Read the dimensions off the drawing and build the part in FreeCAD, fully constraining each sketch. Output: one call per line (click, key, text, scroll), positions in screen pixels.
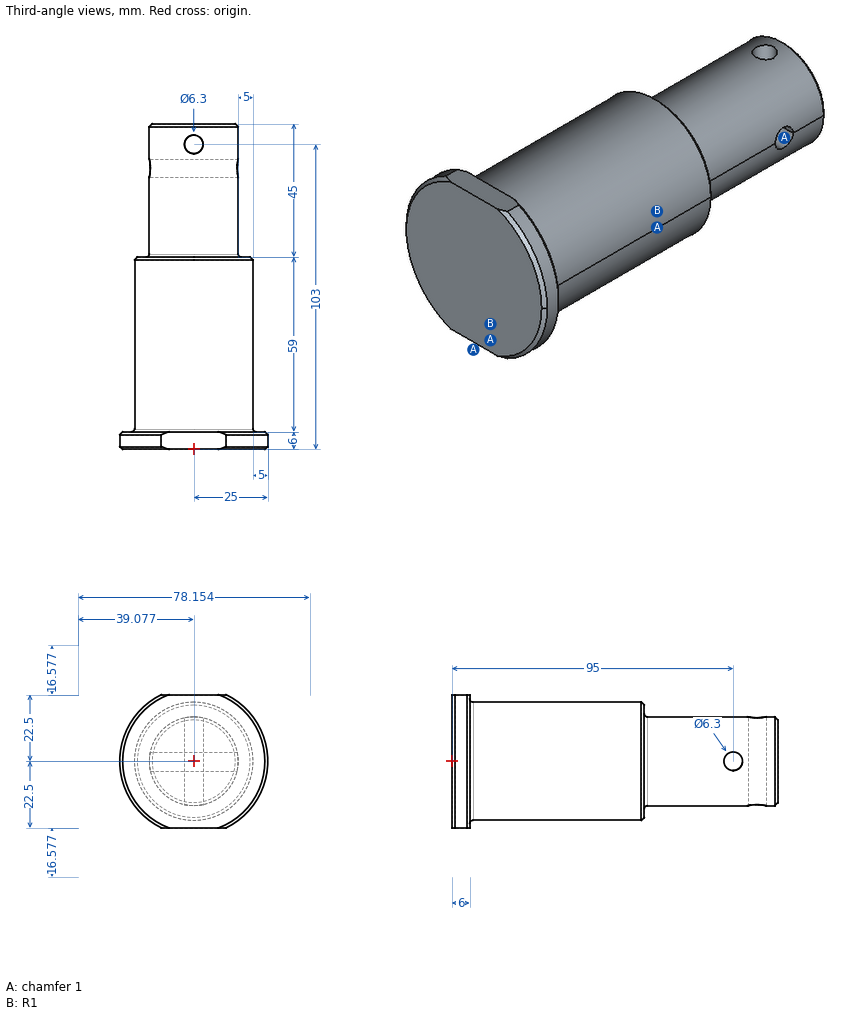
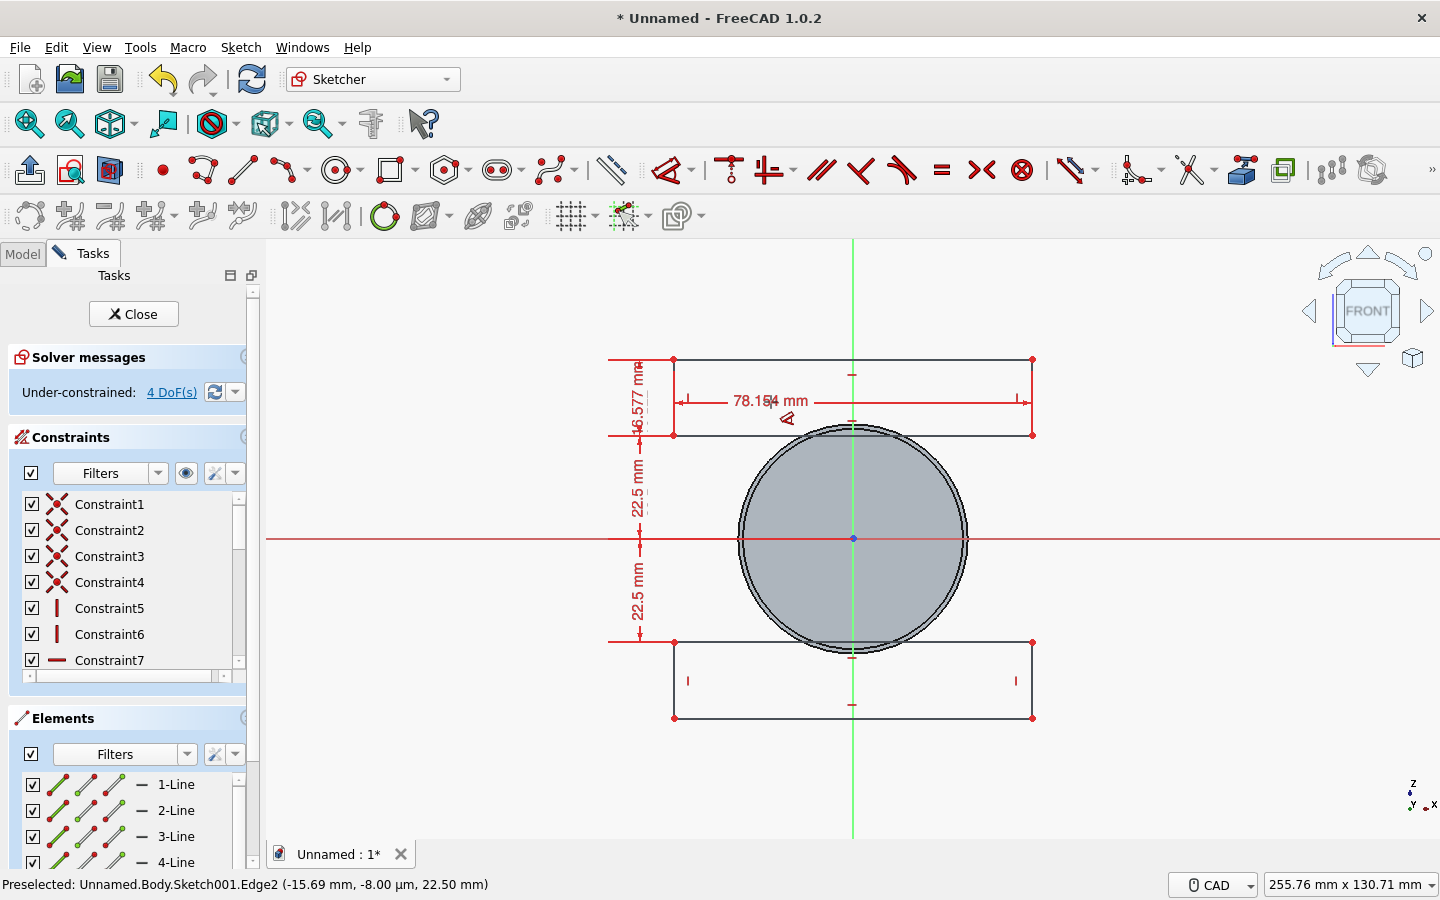
click(674, 665)
click(640, 681)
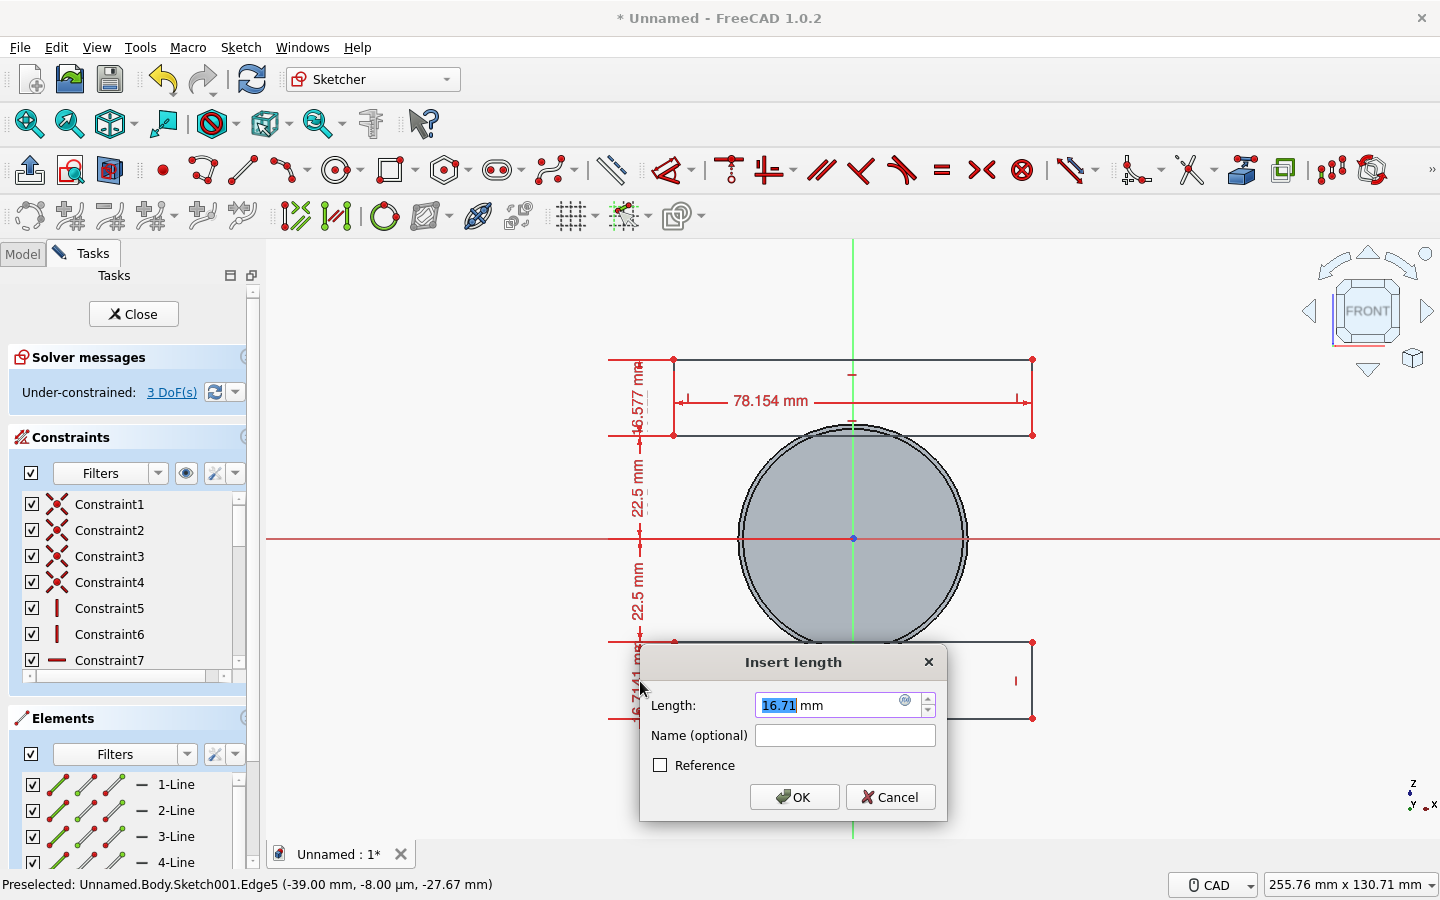
text(16.577)
key(Return)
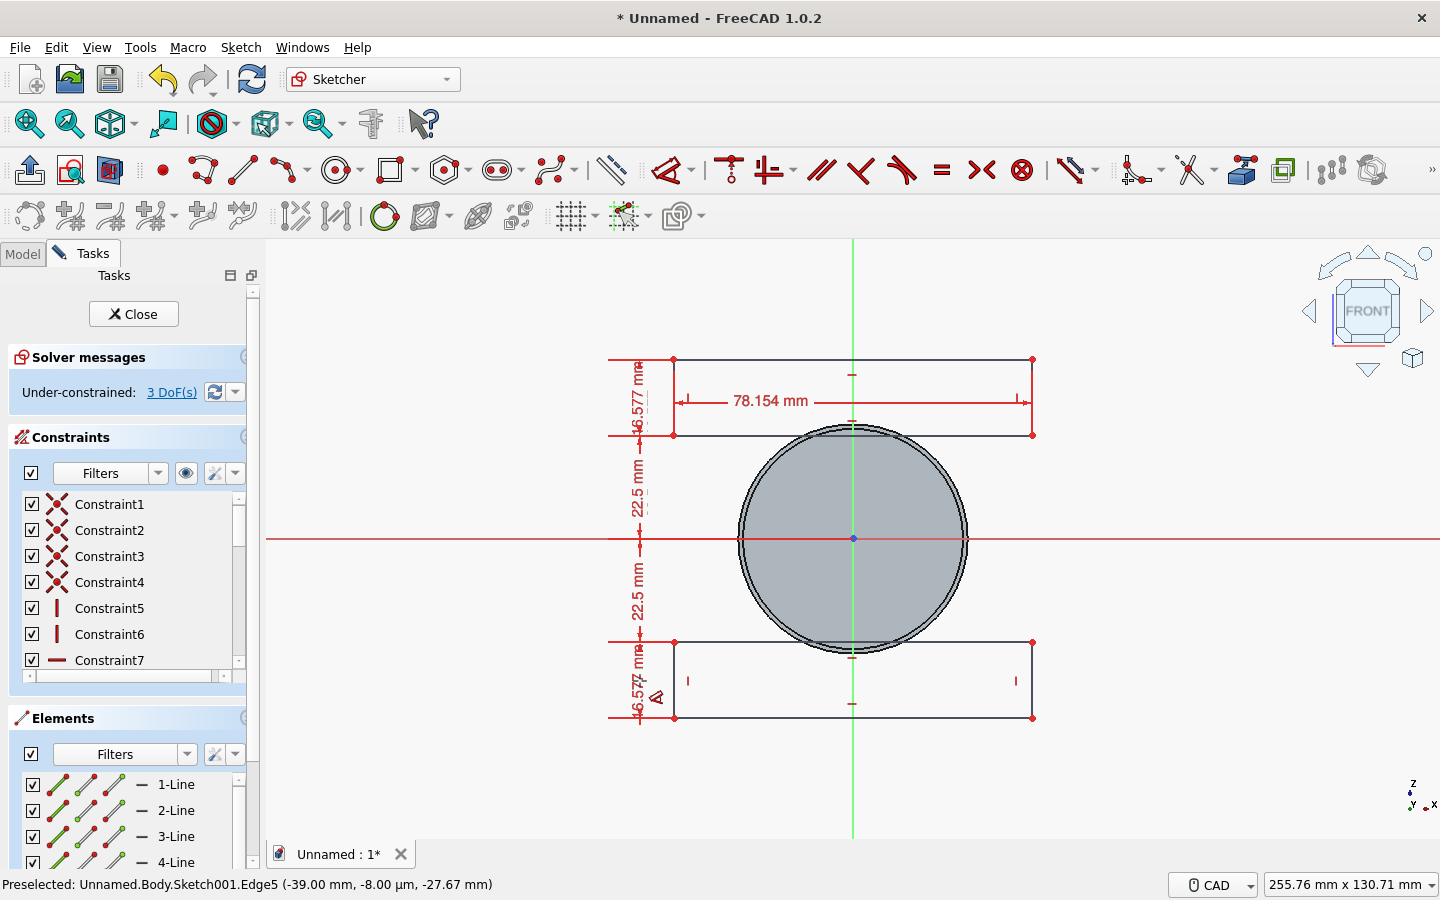
click(781, 718)
click(771, 752)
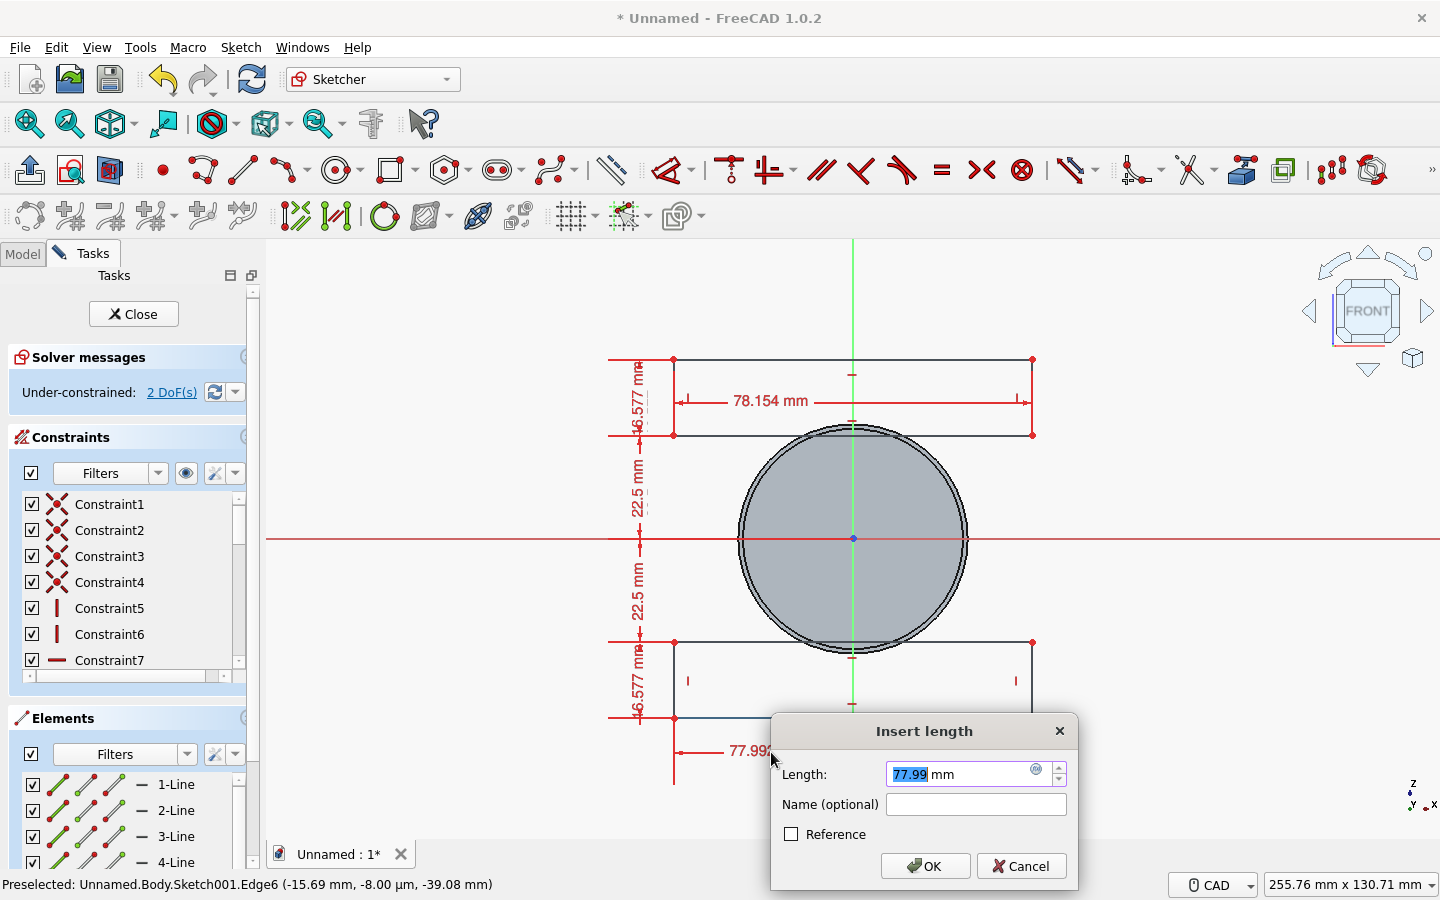
text(78.154)
key(Return)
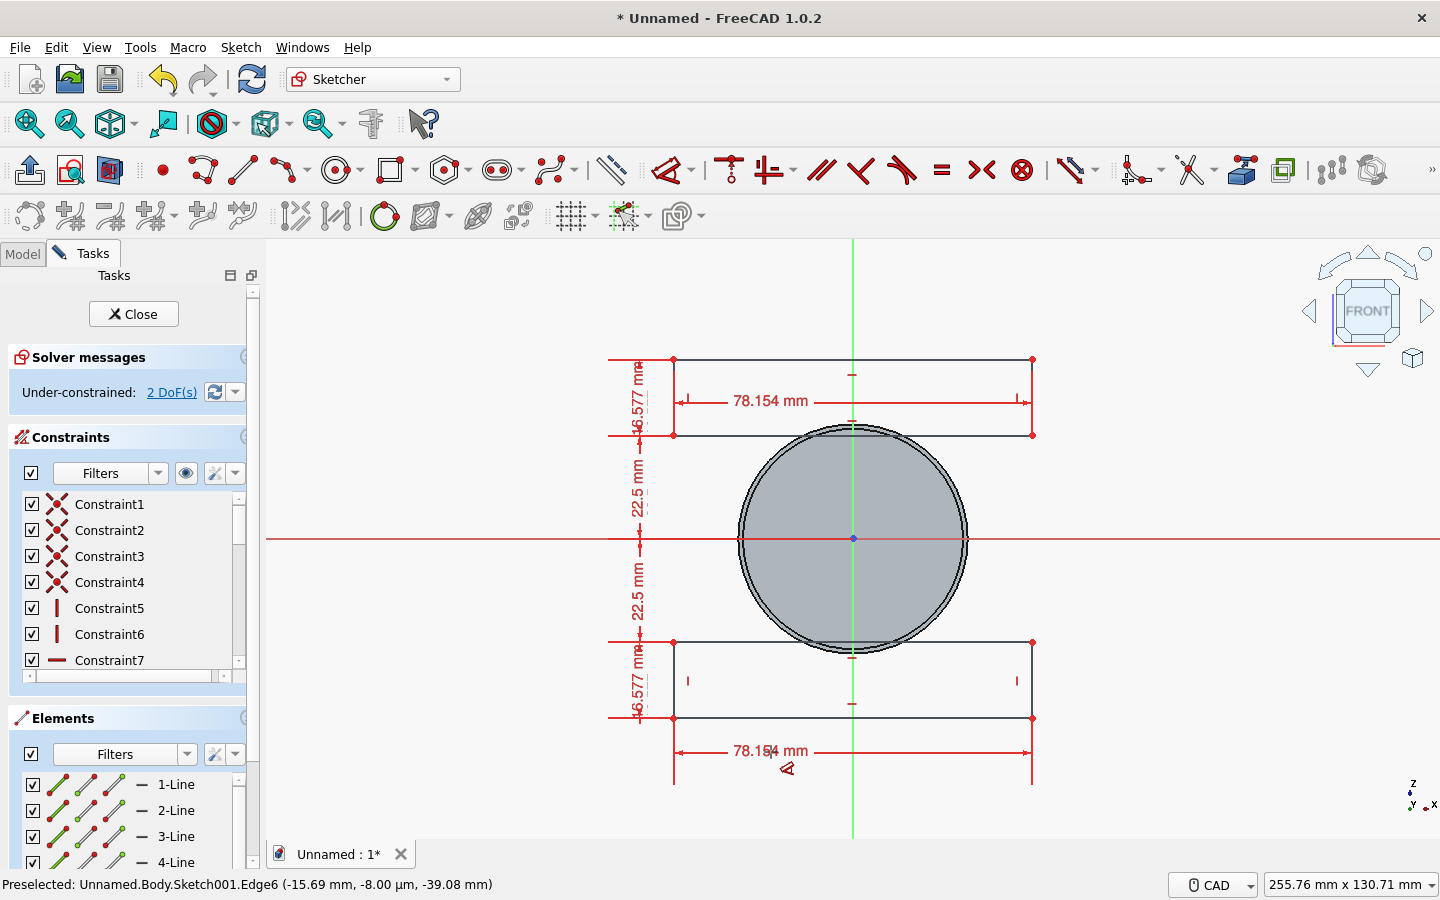
click(674, 360)
click(763, 326)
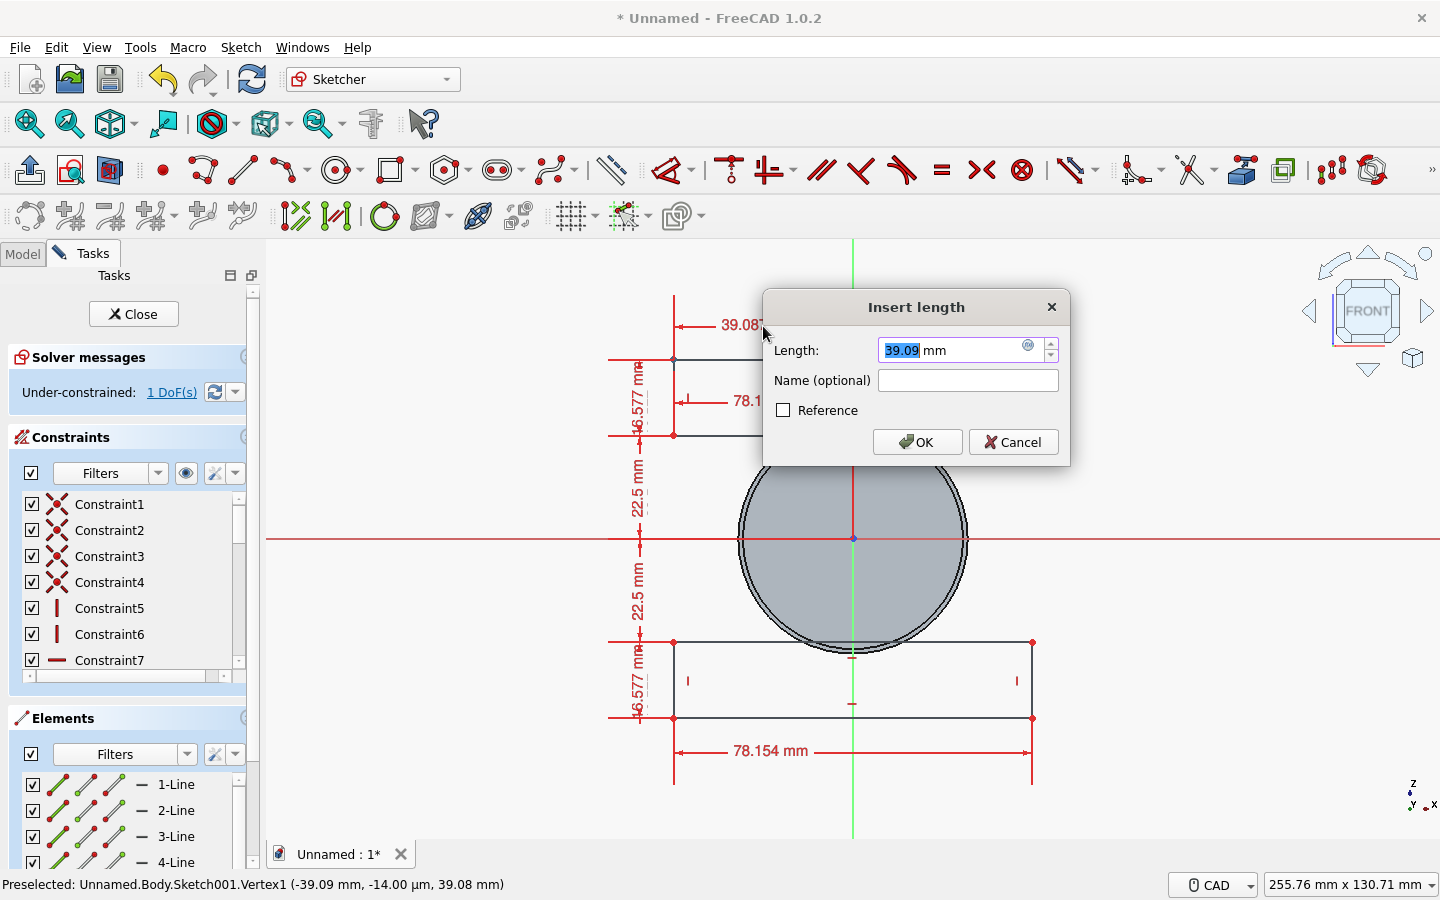
text(39.077)
key(Return)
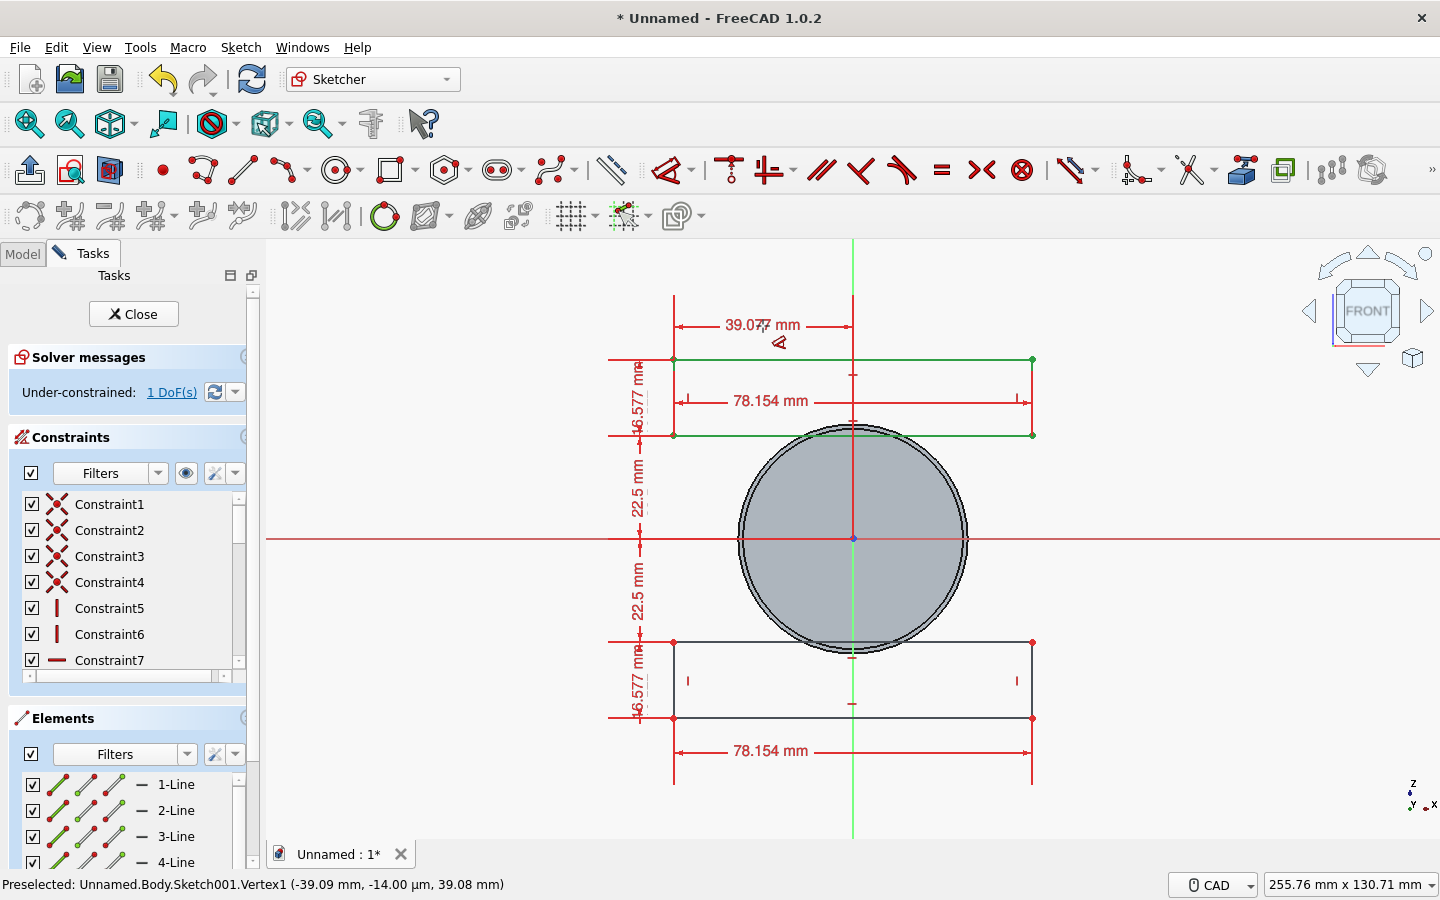
click(674, 642)
click(763, 676)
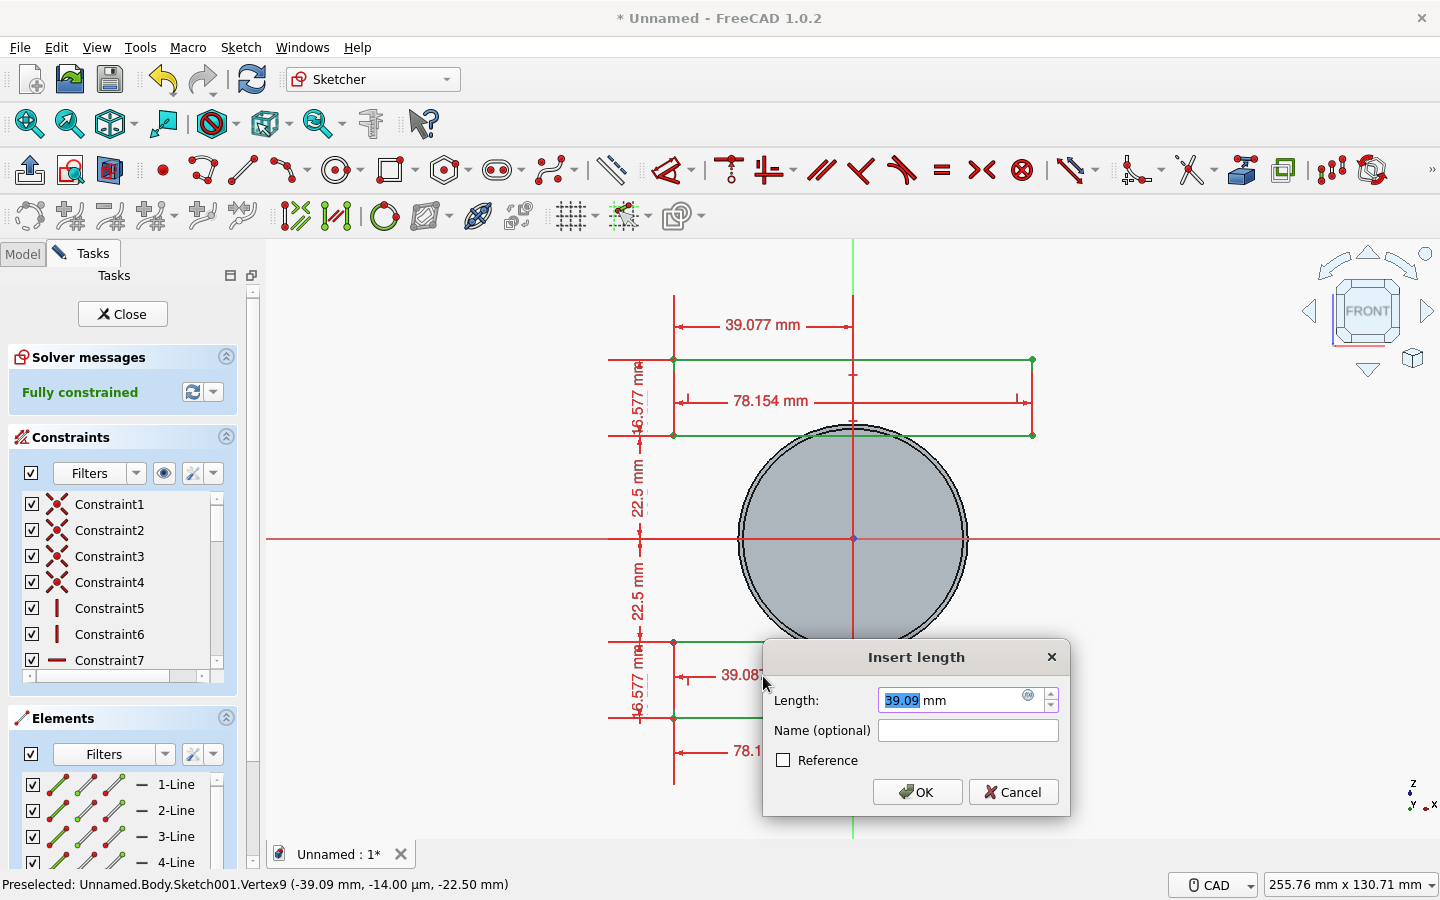
text(39.077)
key(Return)
key(Escape)